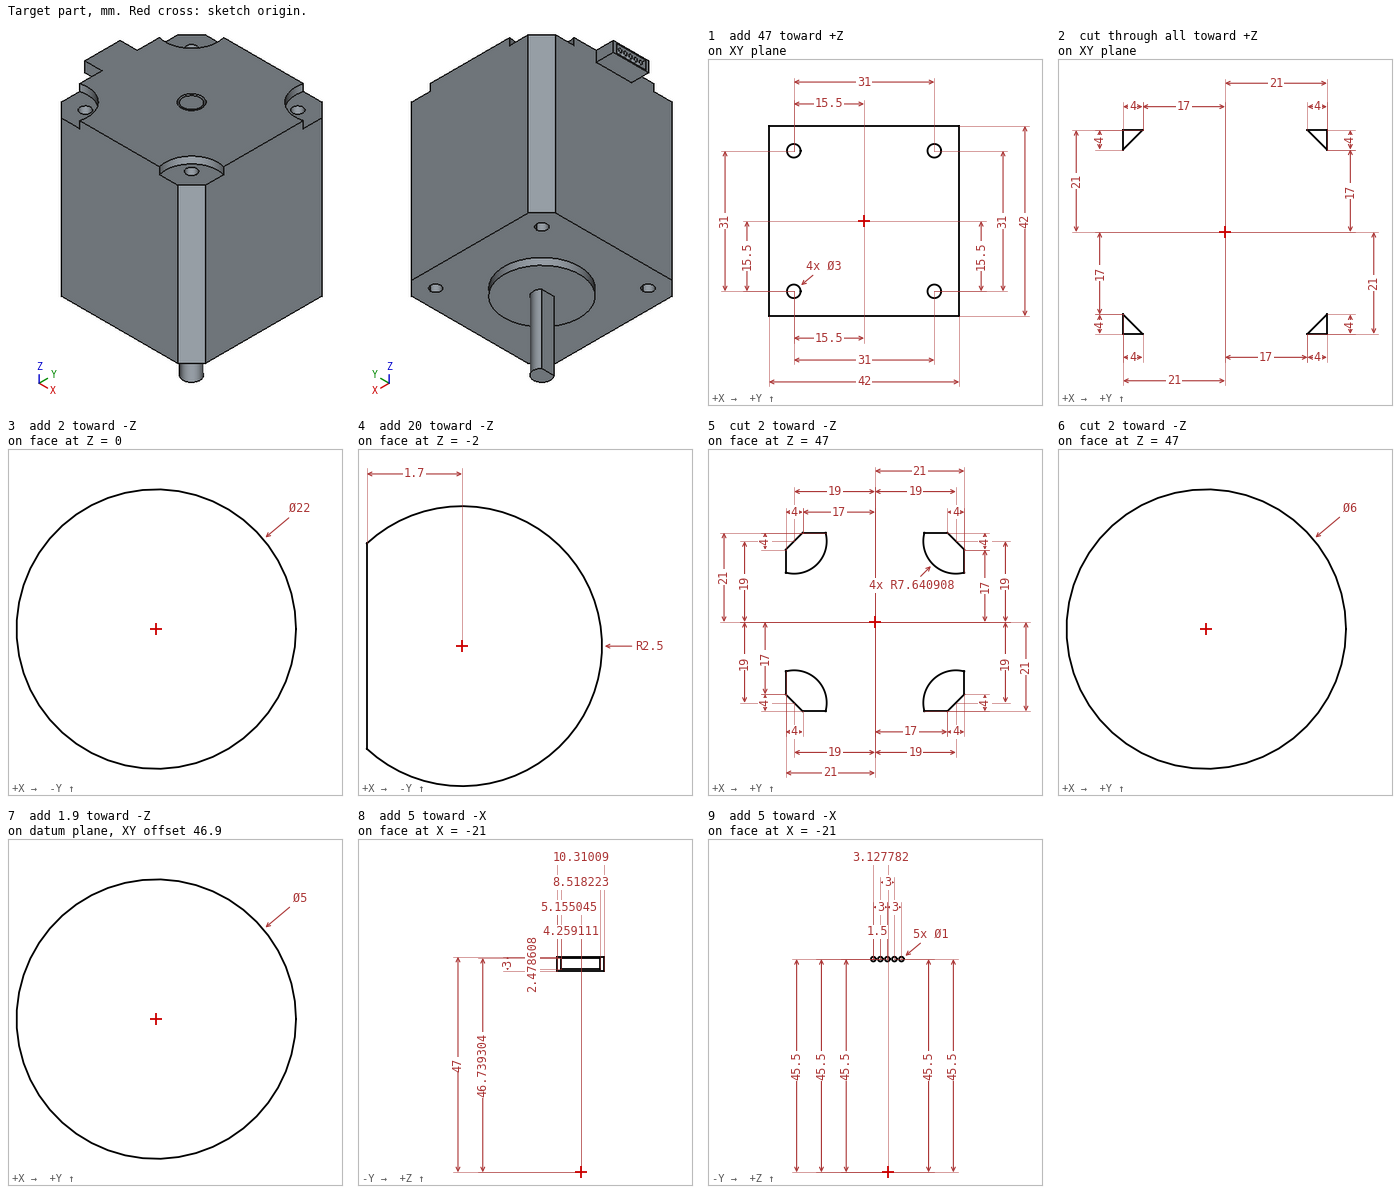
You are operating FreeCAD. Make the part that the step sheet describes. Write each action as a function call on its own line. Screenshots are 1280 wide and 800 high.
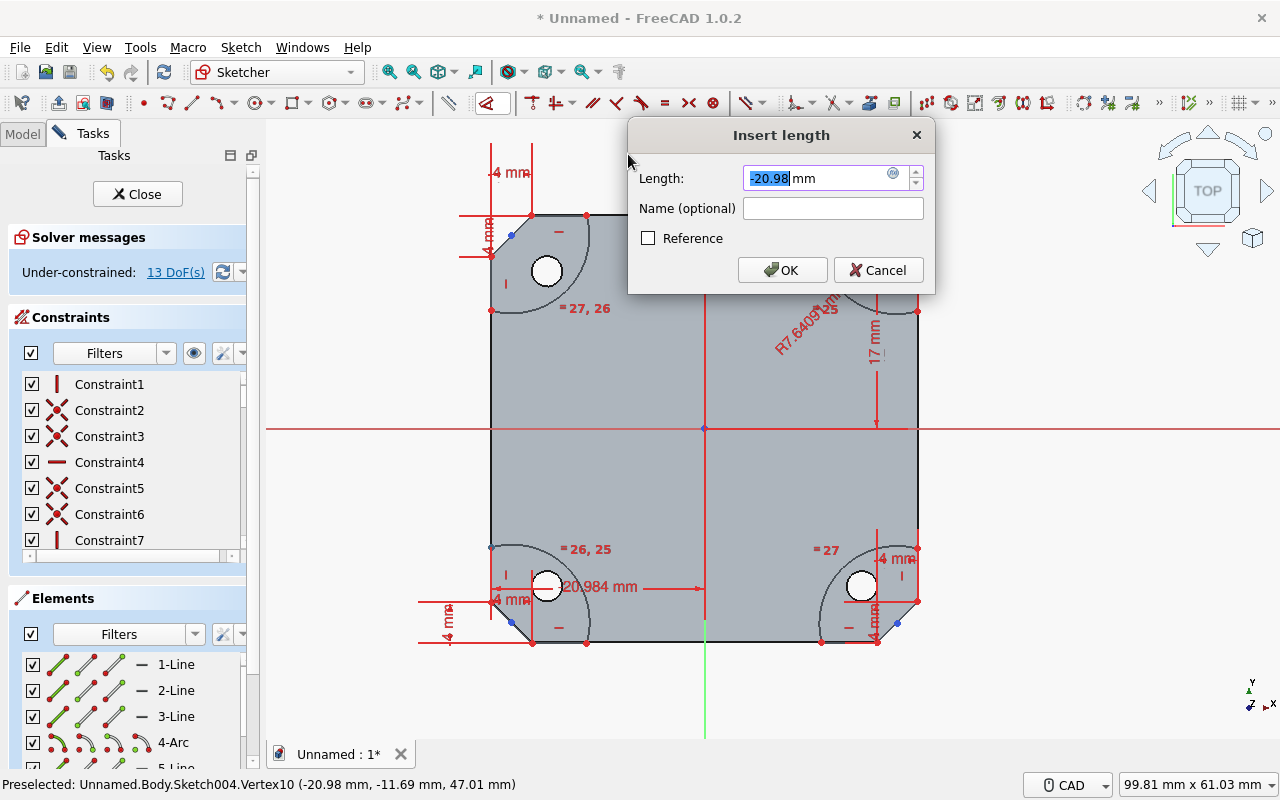
text(-21)
key(Return)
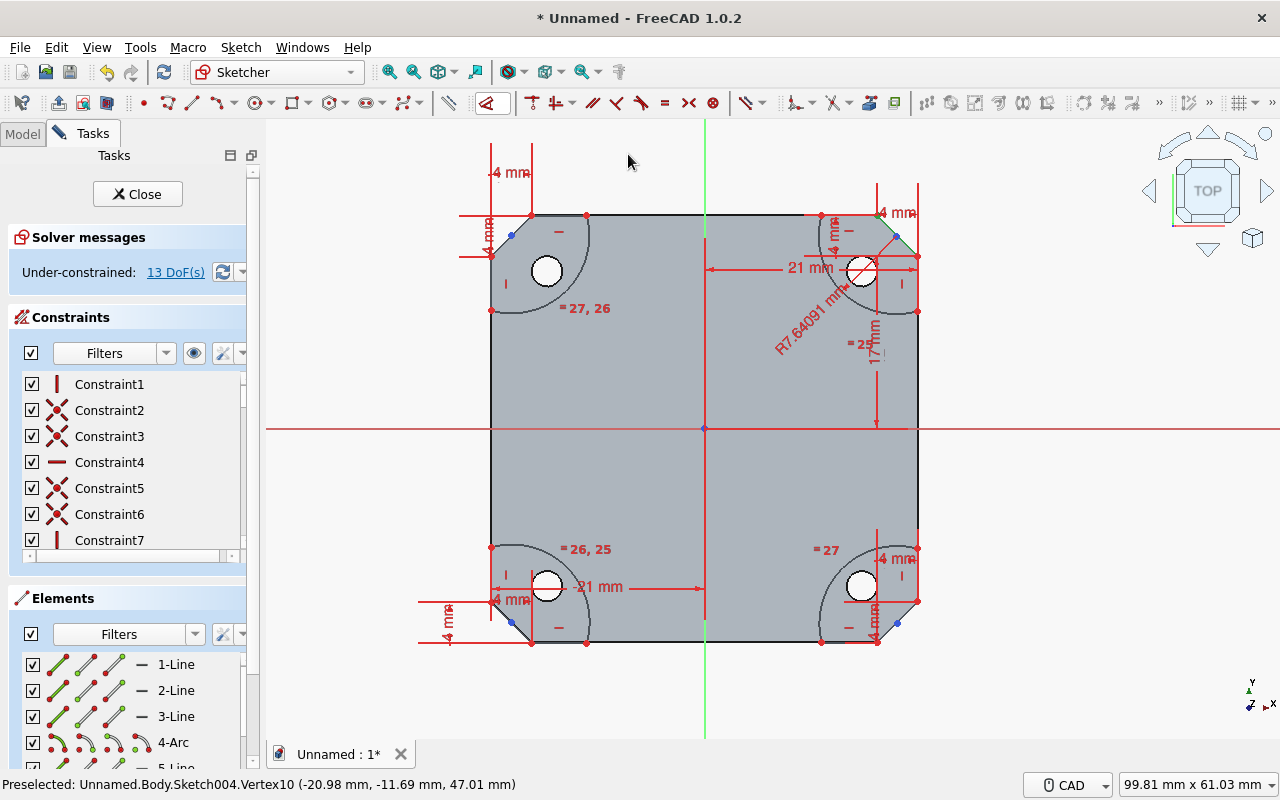
click(491, 602)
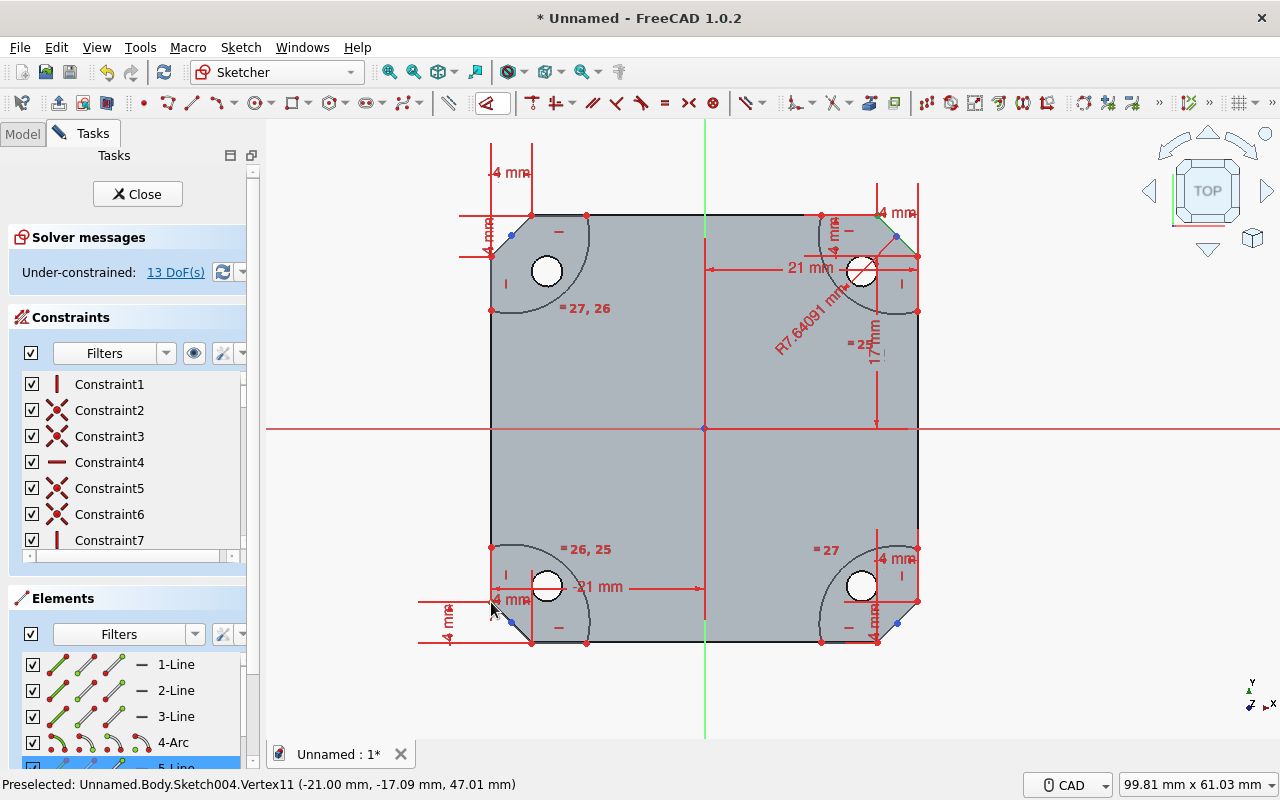
key(i)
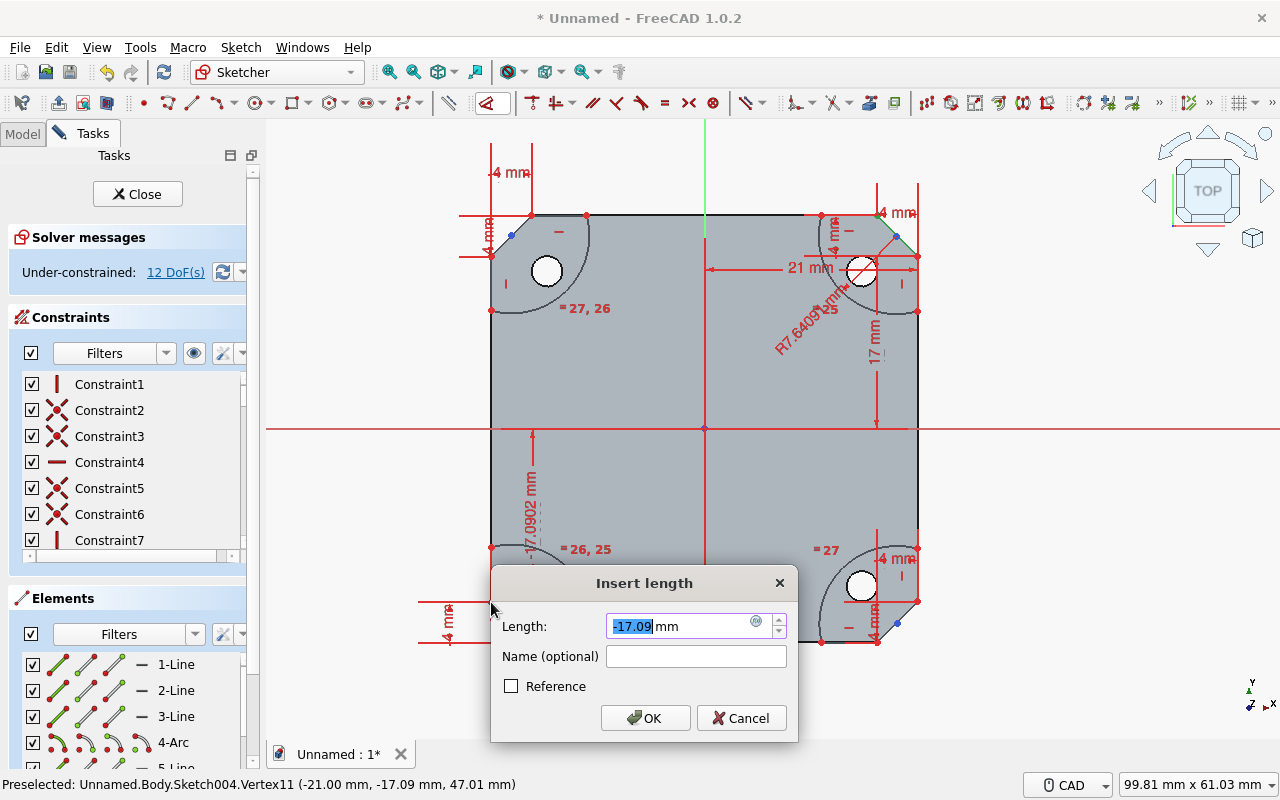
text(-17)
key(Return)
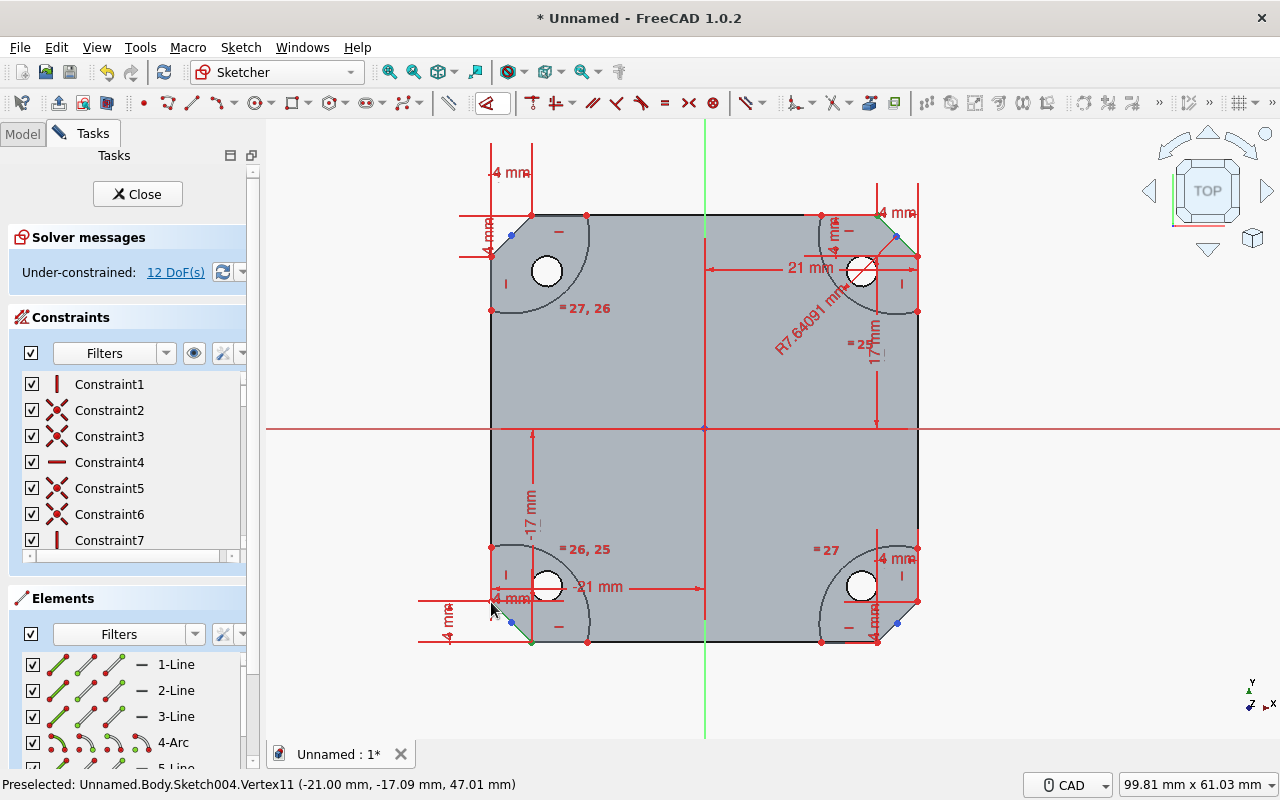
click(587, 216)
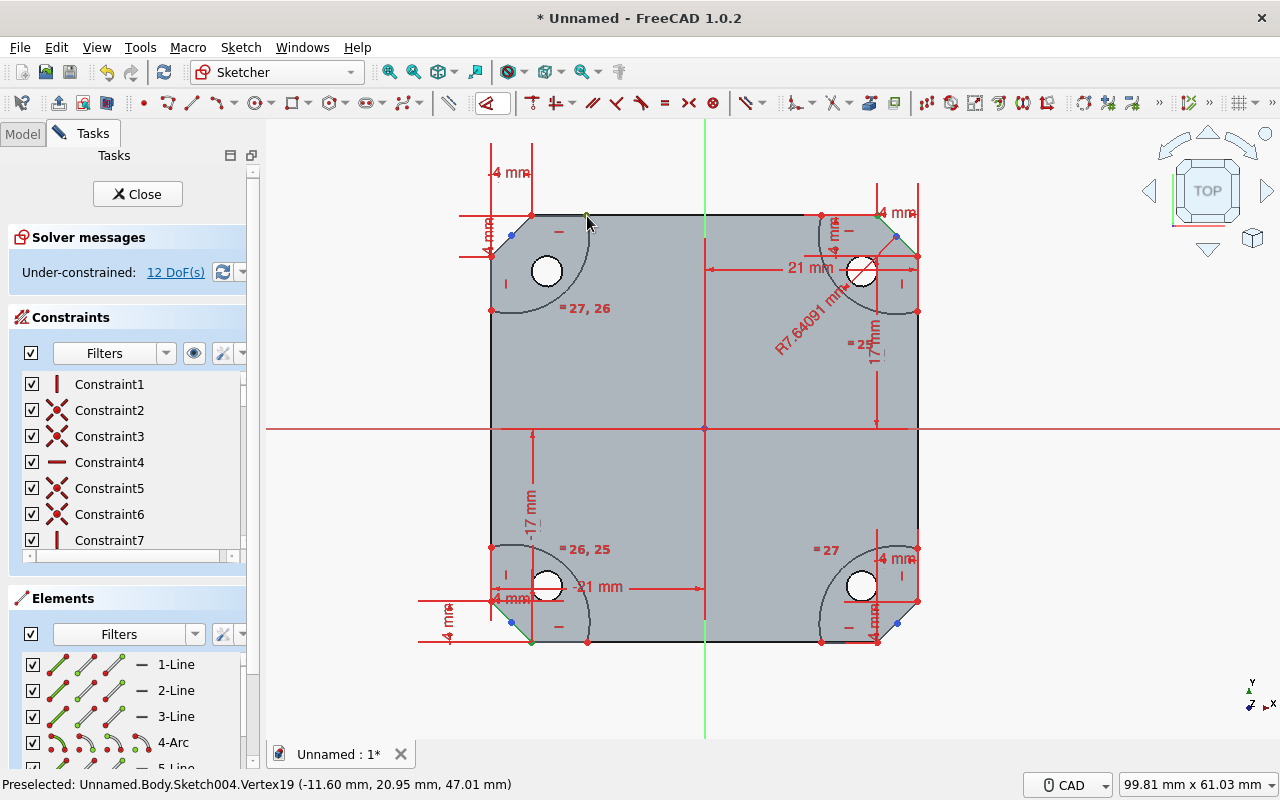
click(504, 104)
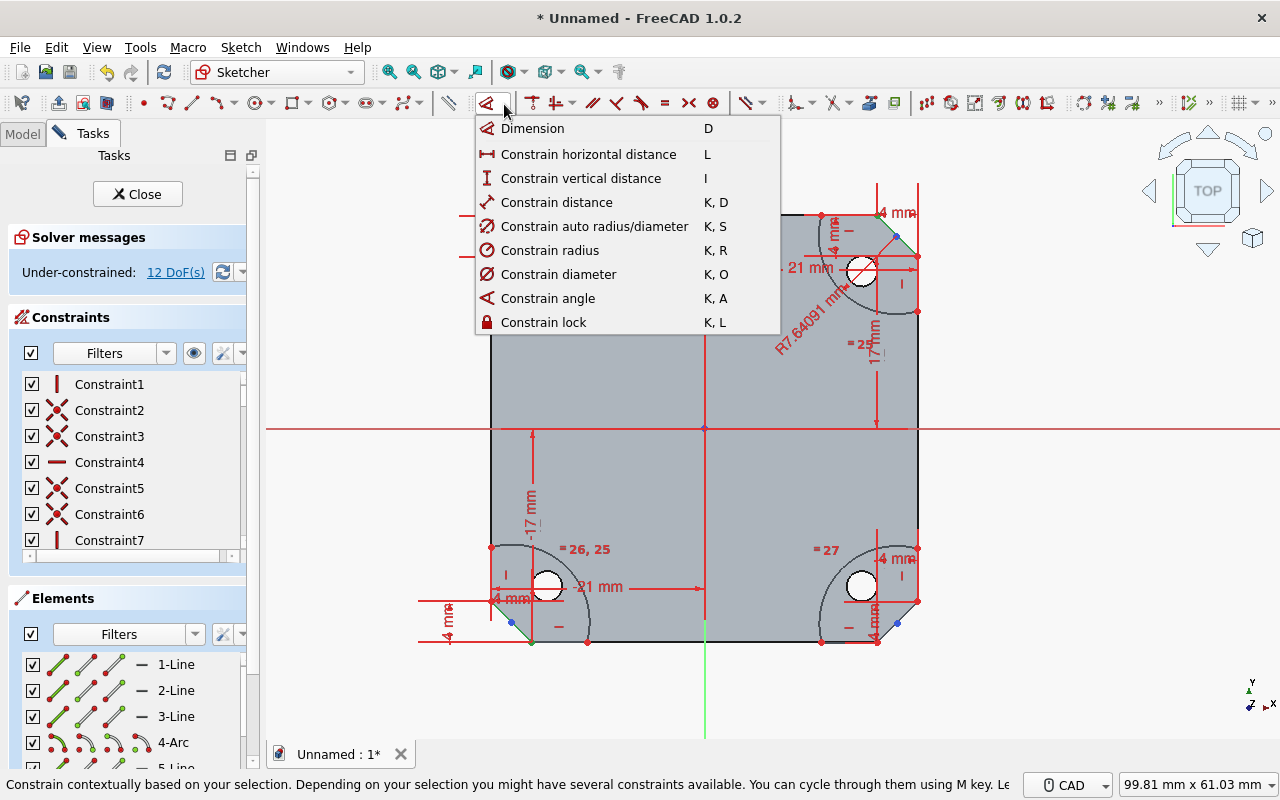
click(628, 178)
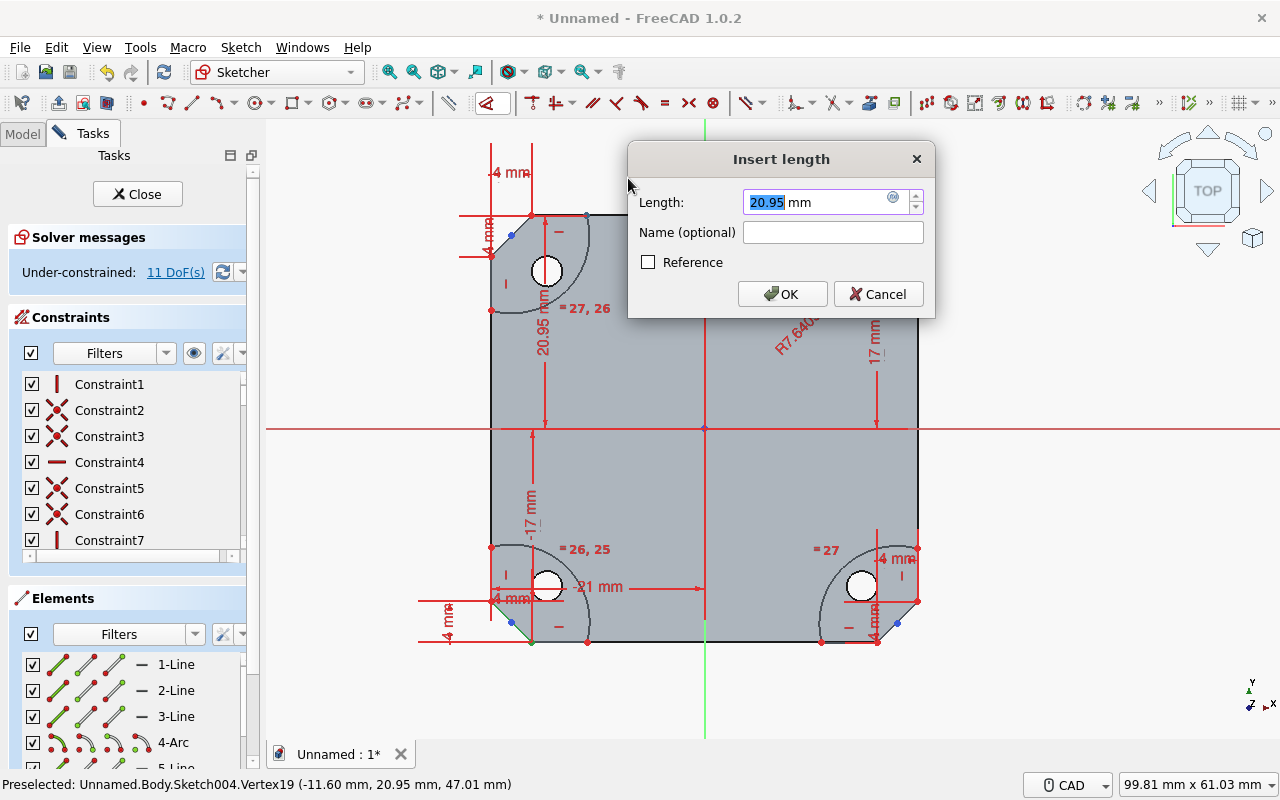
text(21)
key(Return)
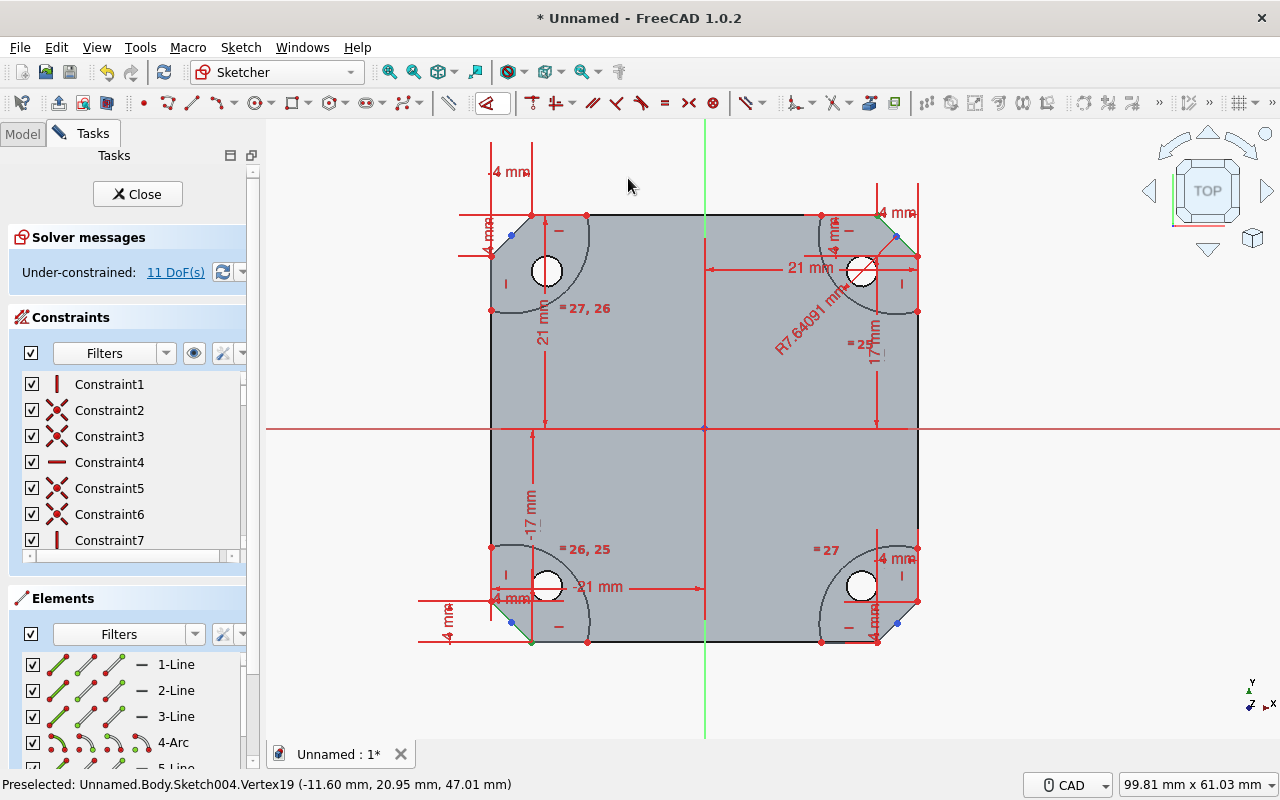
click(532, 215)